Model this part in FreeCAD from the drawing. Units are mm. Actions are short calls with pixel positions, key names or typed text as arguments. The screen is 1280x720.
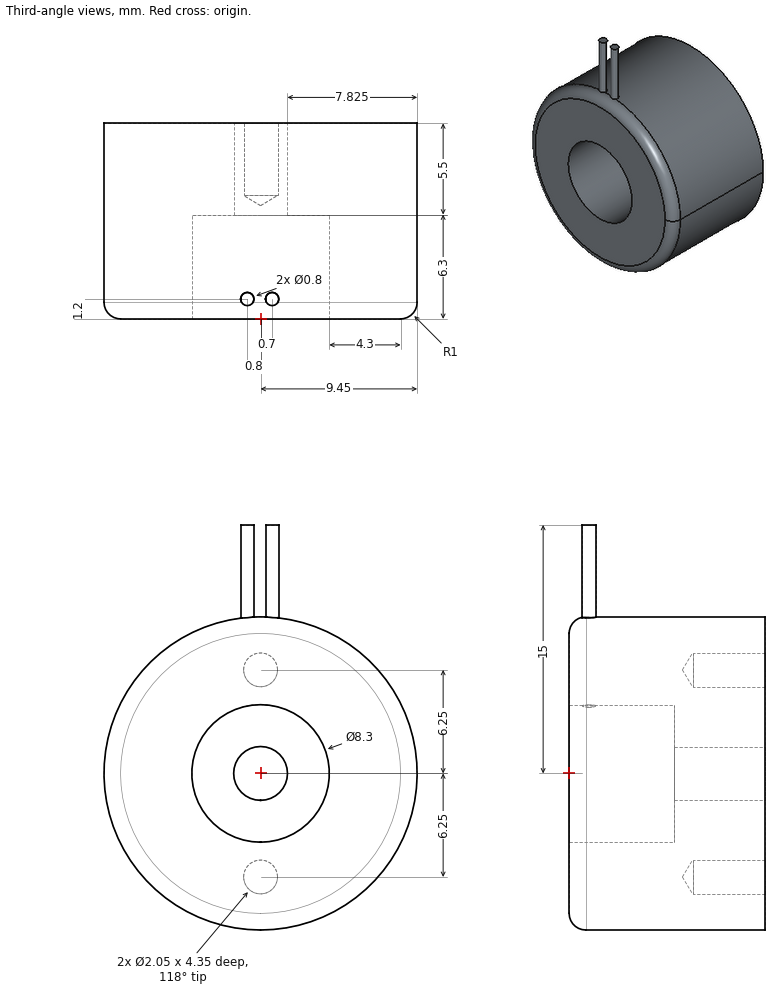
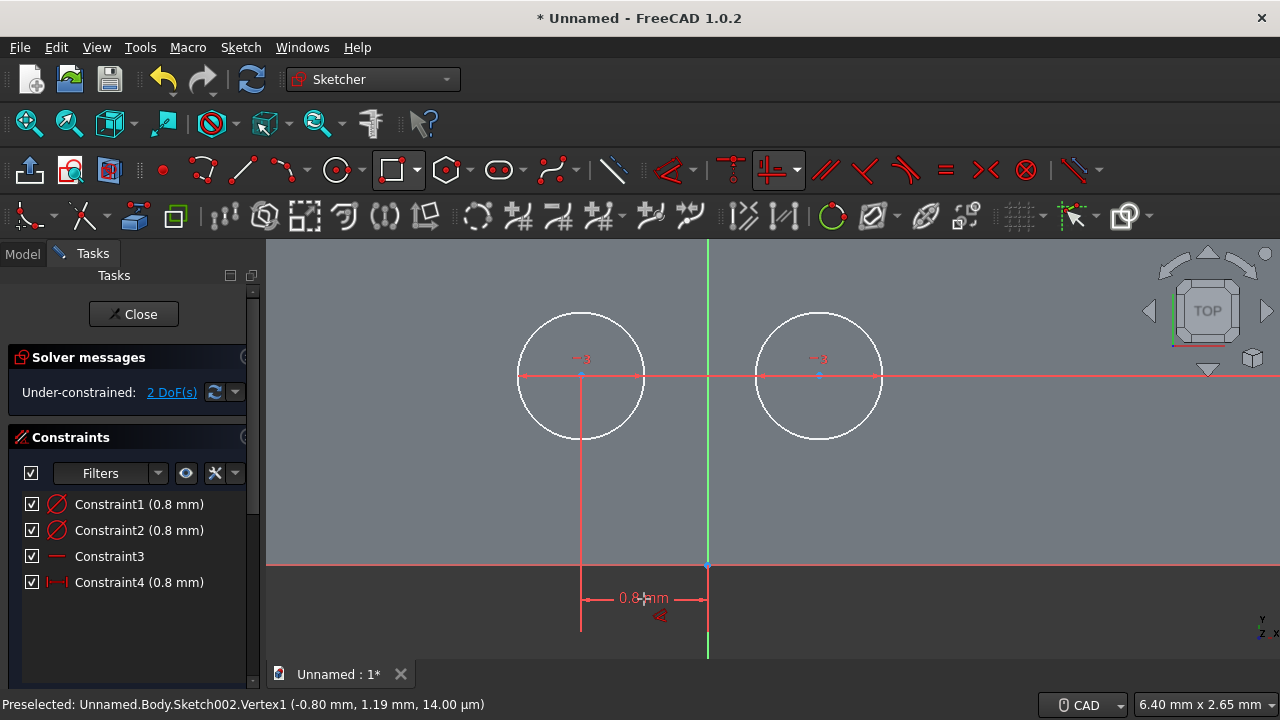
click(581, 376)
click(547, 471)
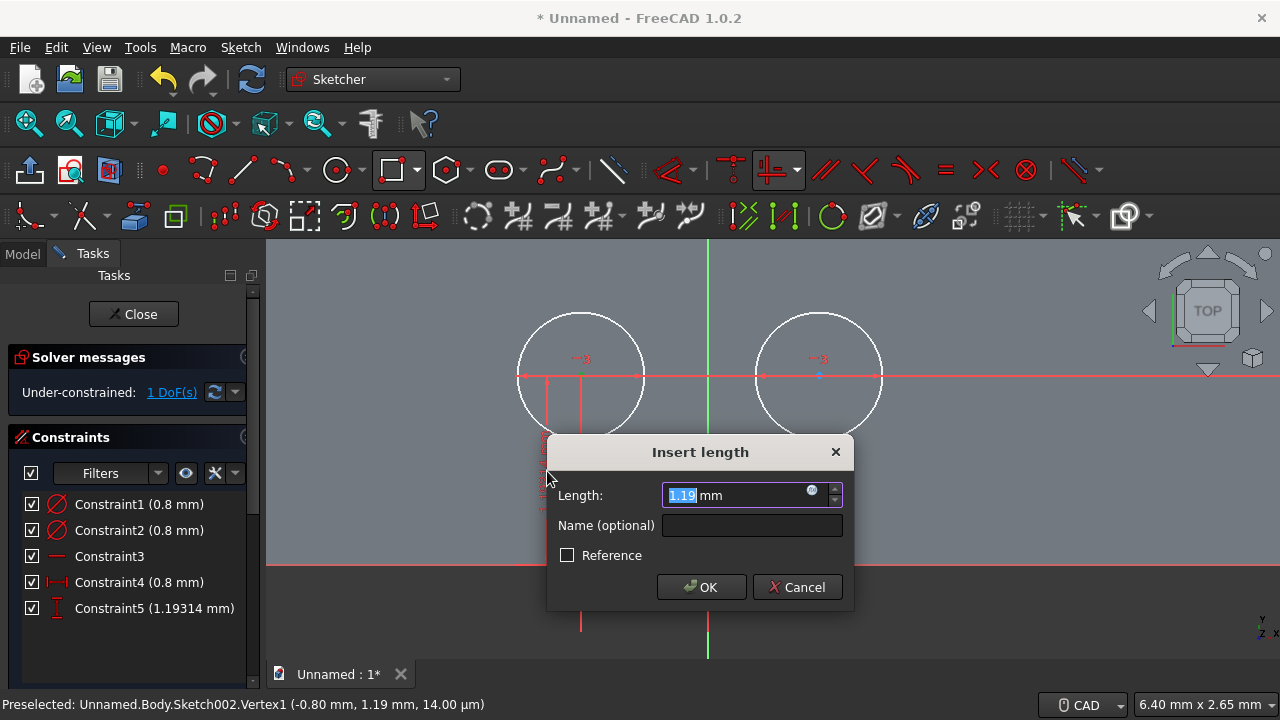
text(1.2)
key(Return)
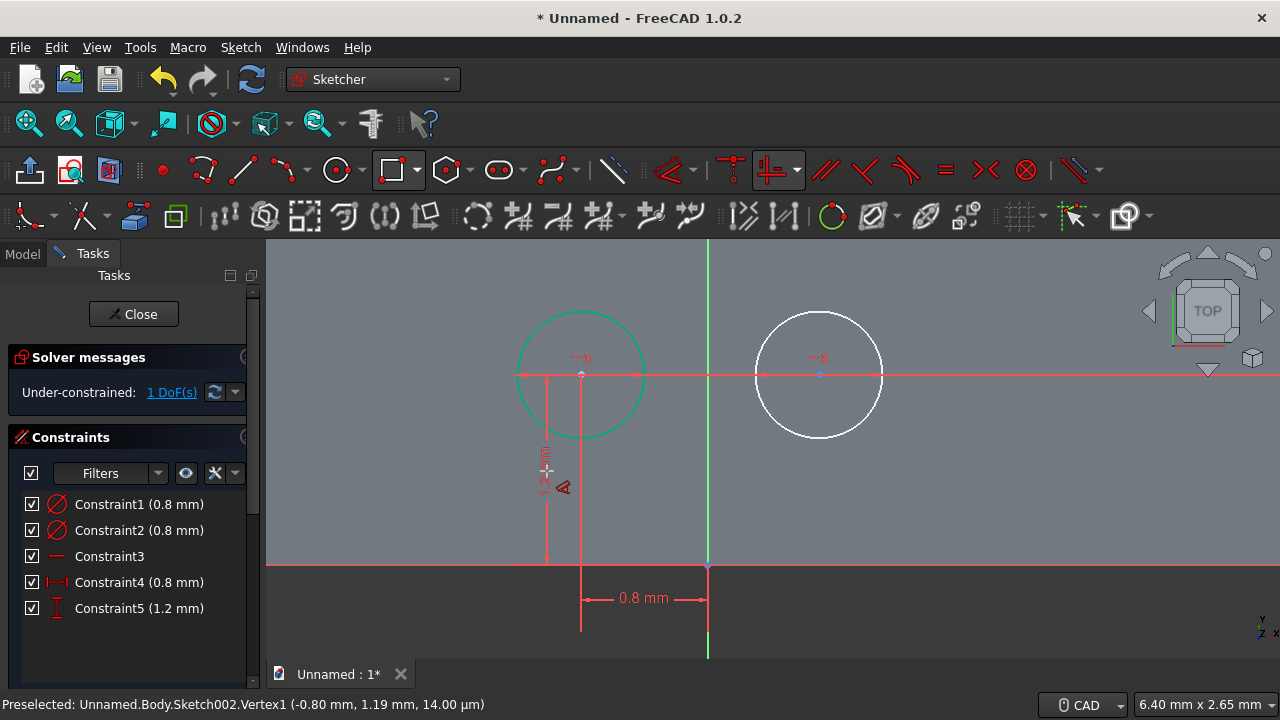
click(819, 375)
click(763, 599)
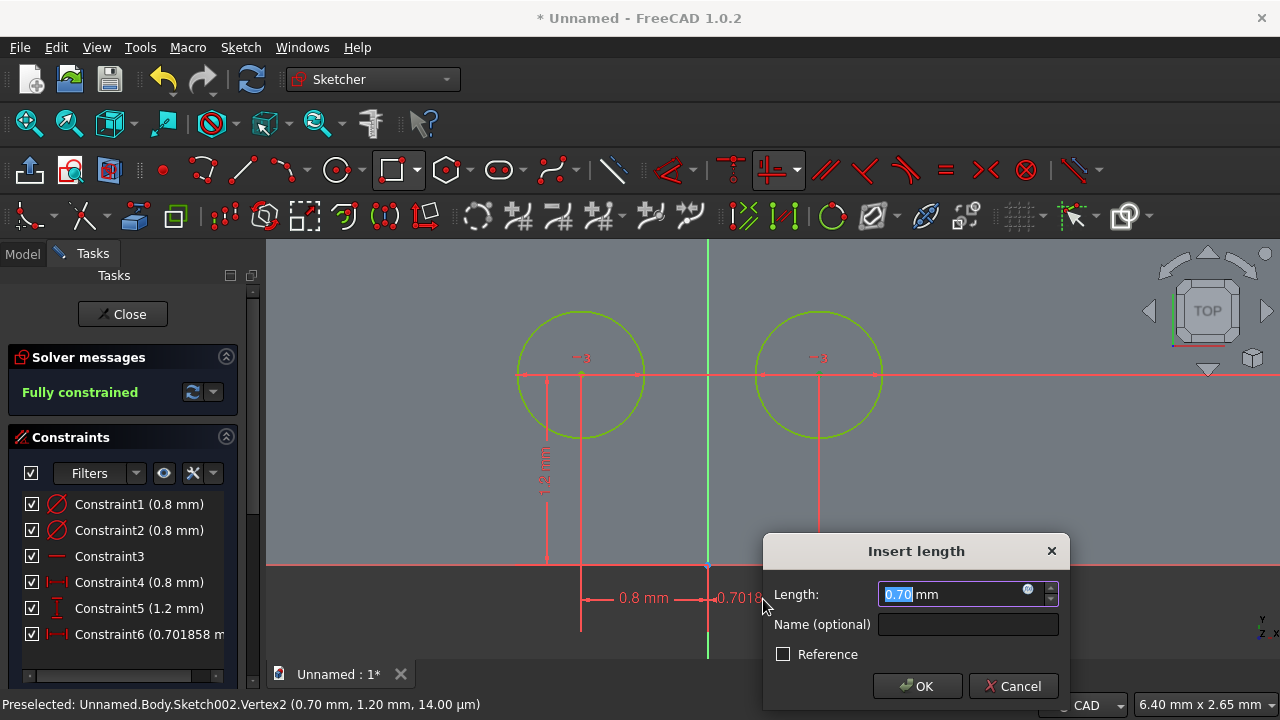
text(0.7)
key(Return)
key(Escape)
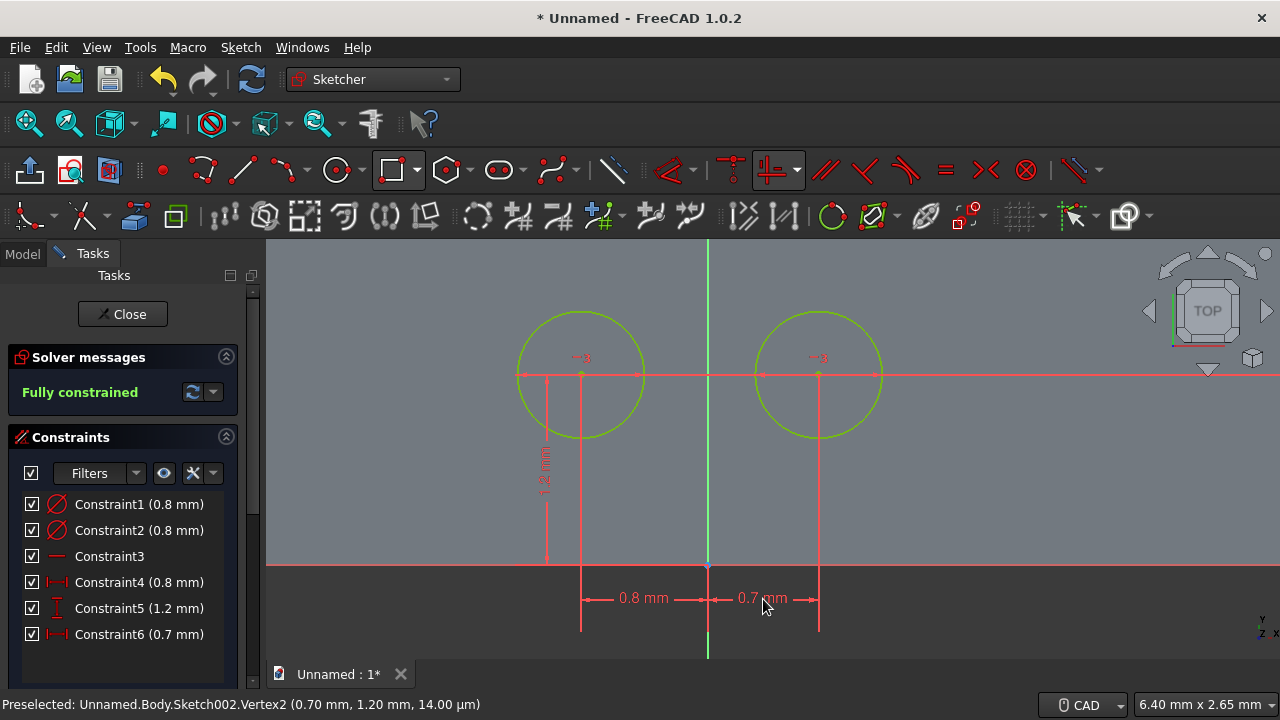
click(123, 314)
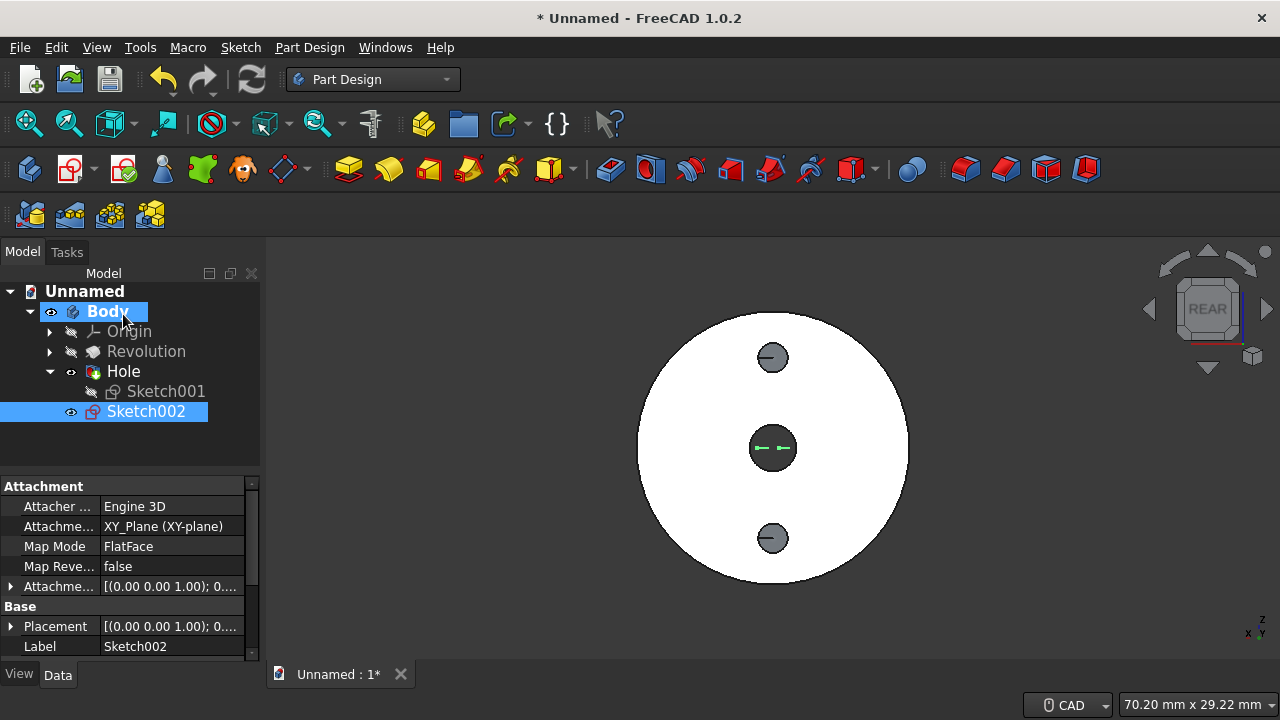
click(350, 170)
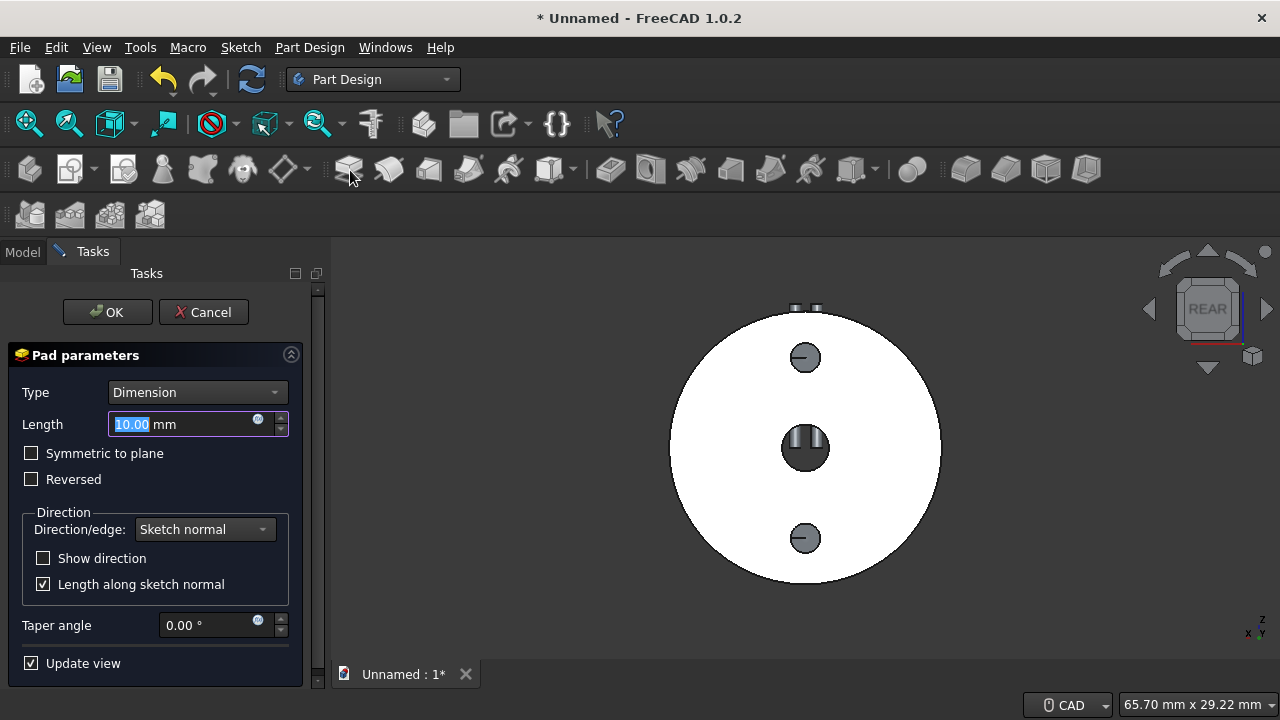
text(15)
key(Tab)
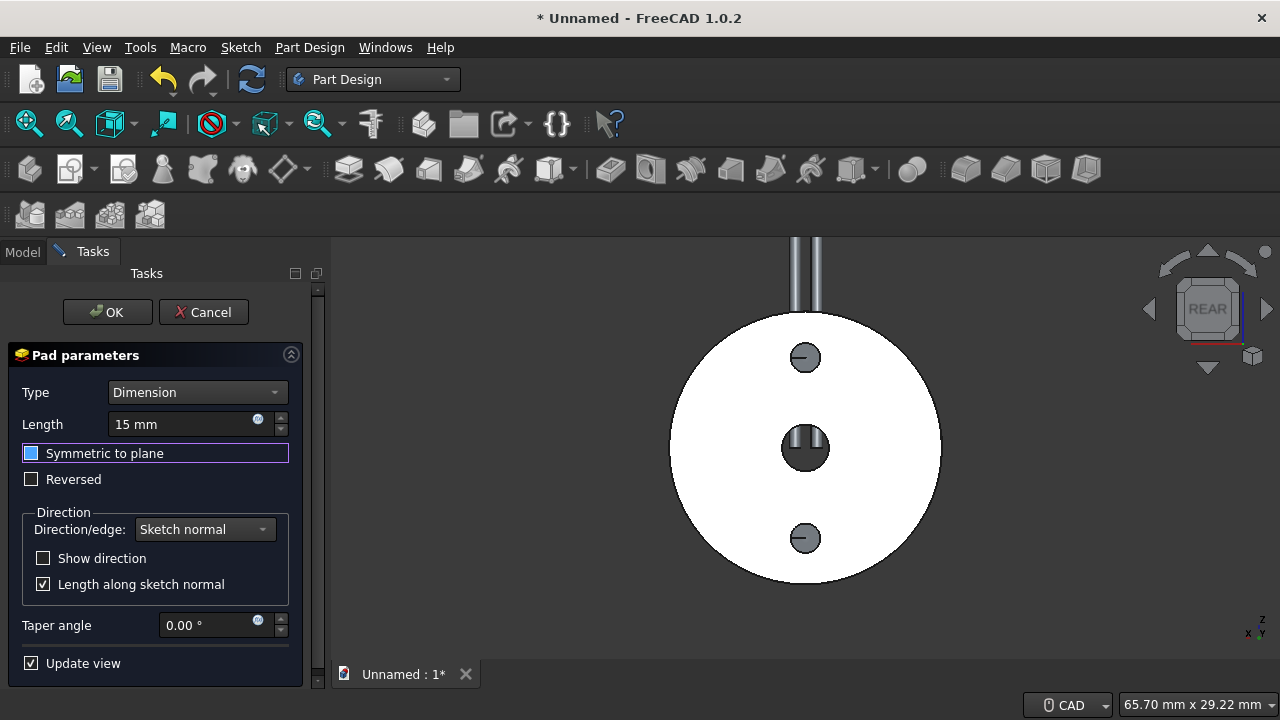
click(108, 312)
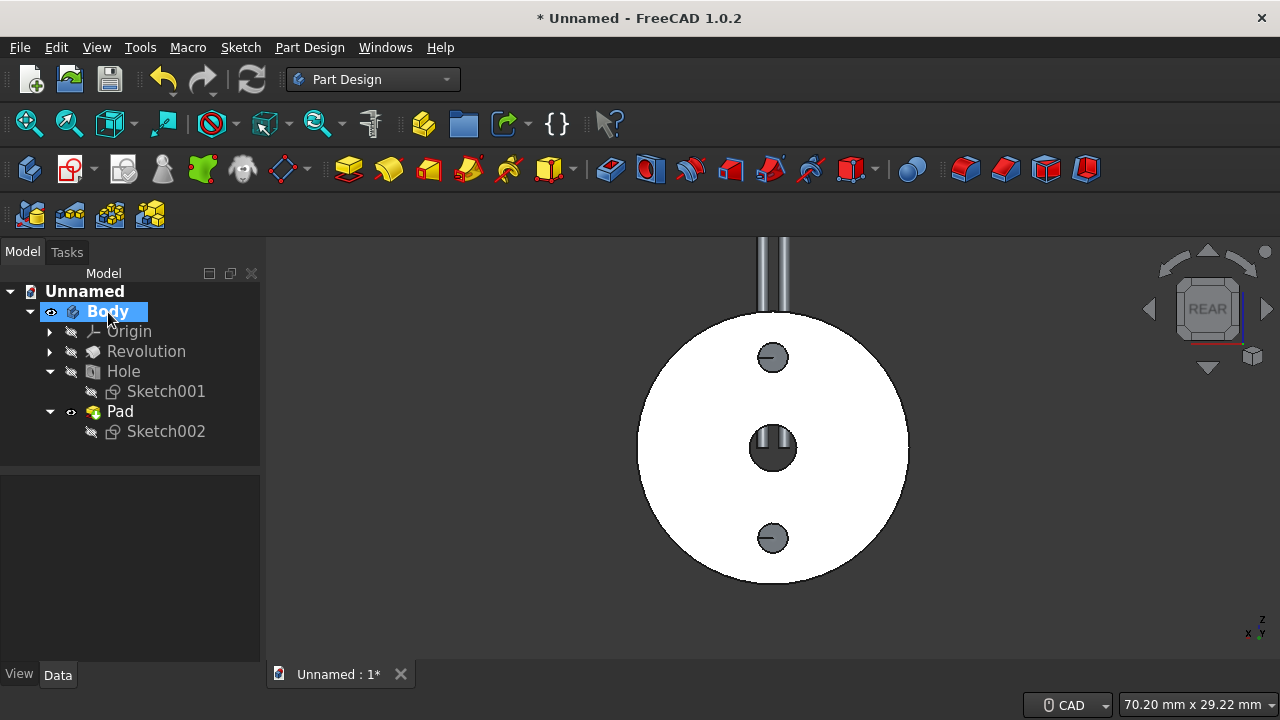
key(v)
key(f)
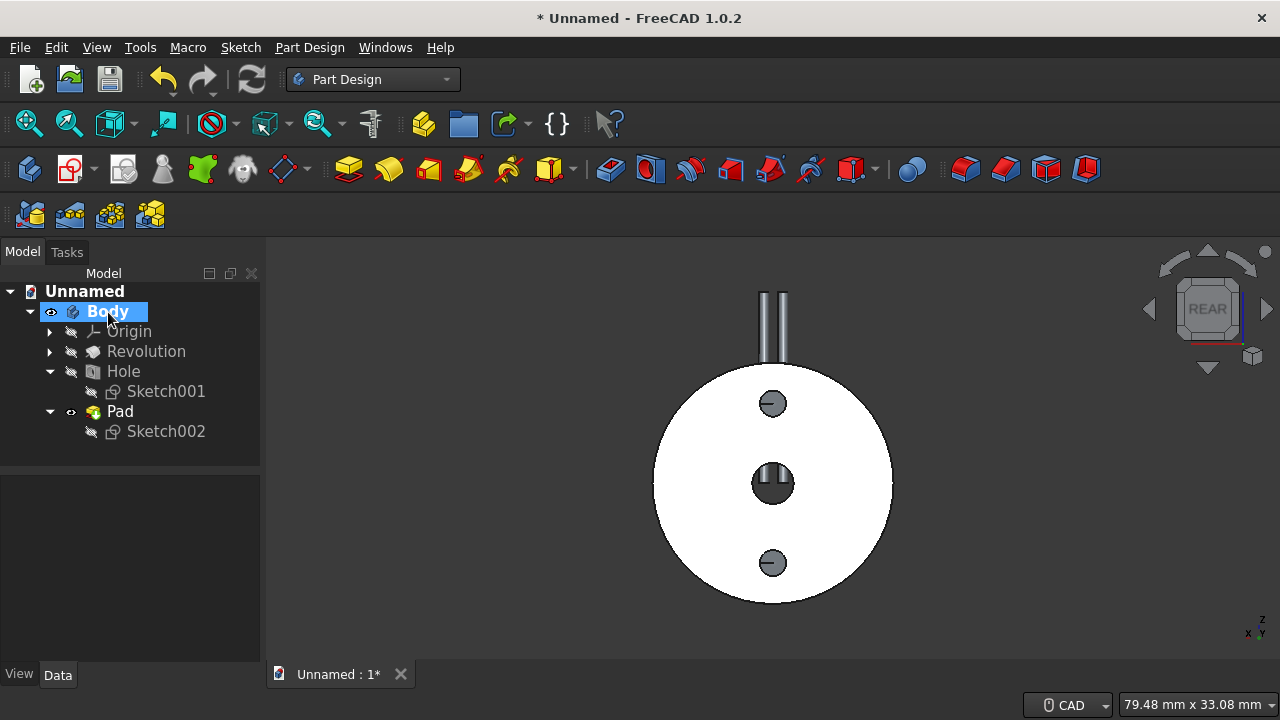
key(0)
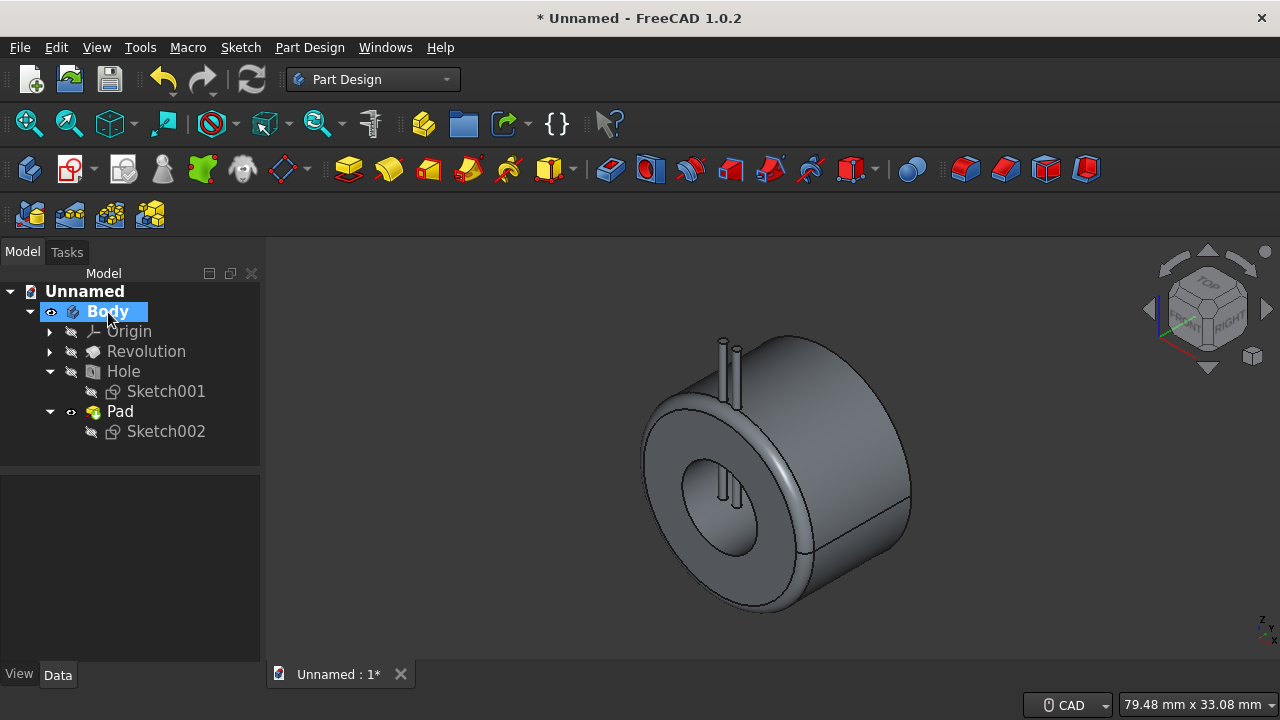
key(1)